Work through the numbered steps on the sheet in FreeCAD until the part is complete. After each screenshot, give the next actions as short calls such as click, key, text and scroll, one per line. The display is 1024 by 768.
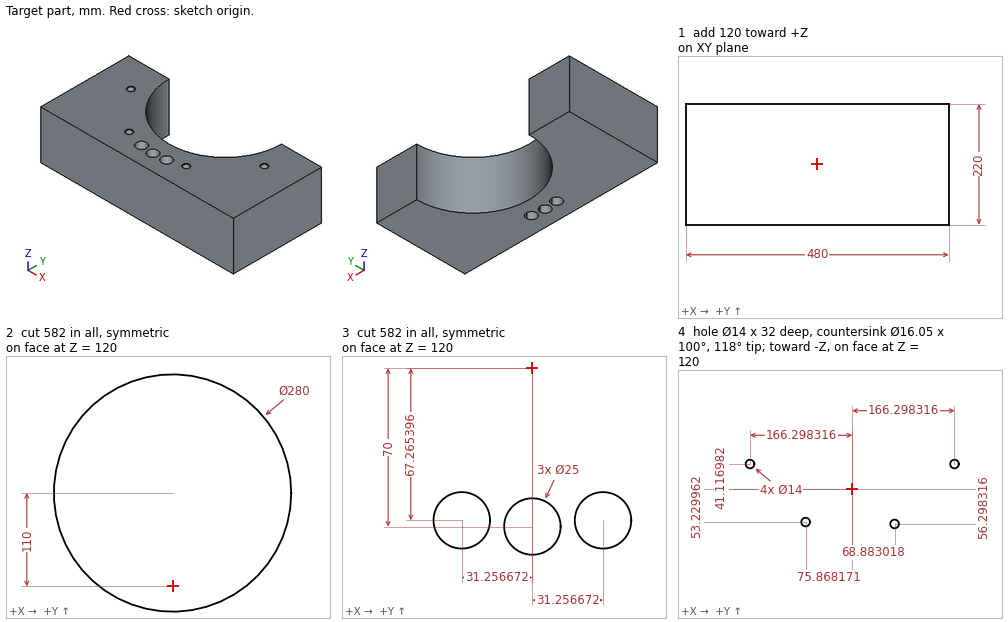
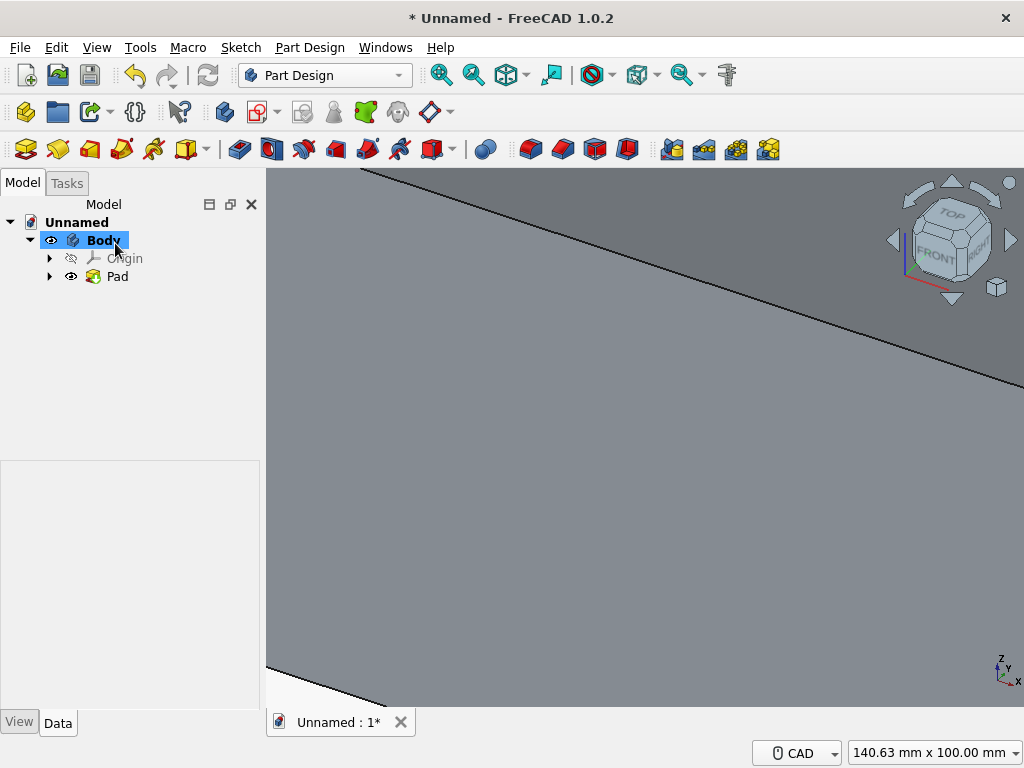
key(v)
key(f)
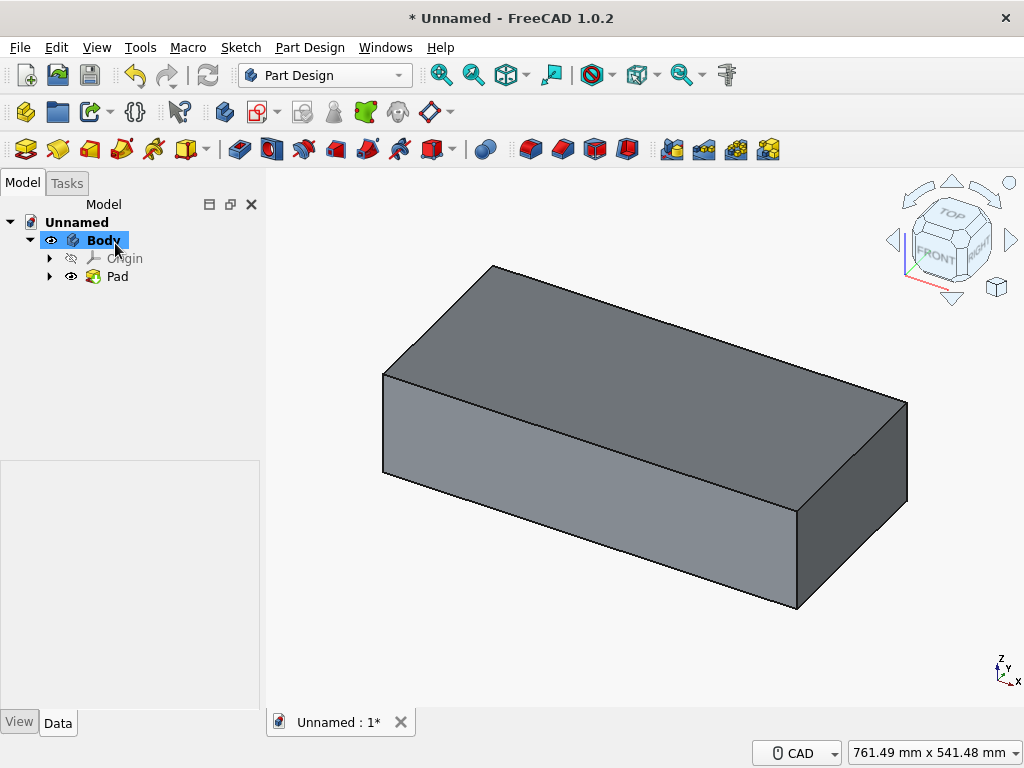
click(704, 407)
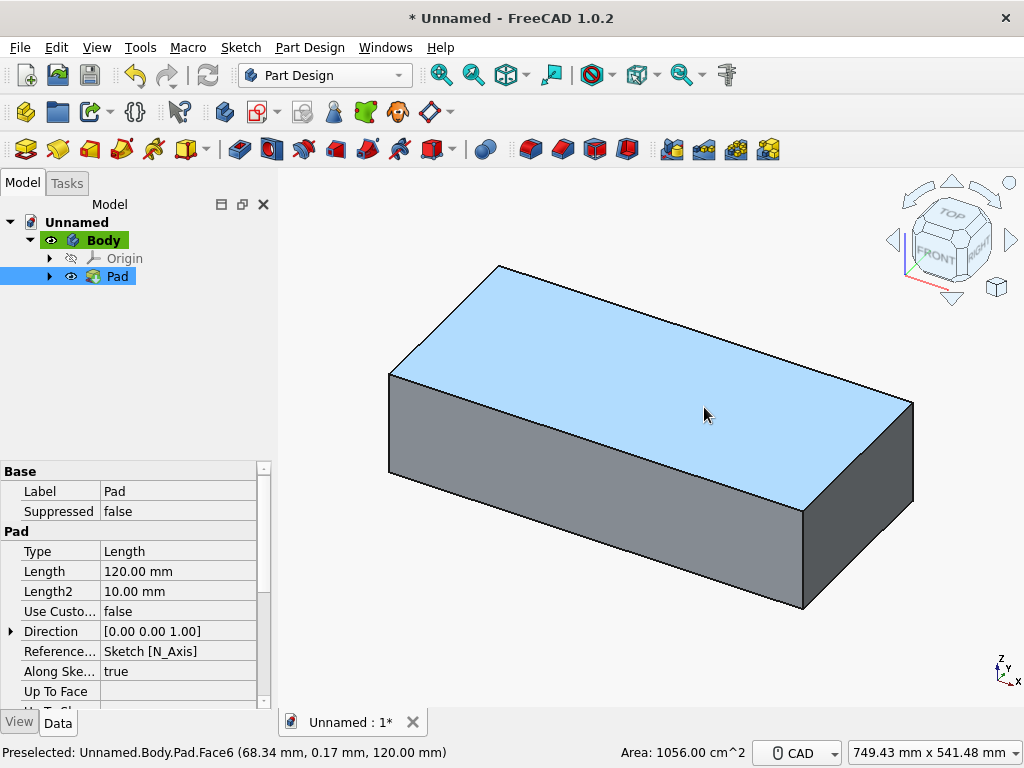
click(258, 112)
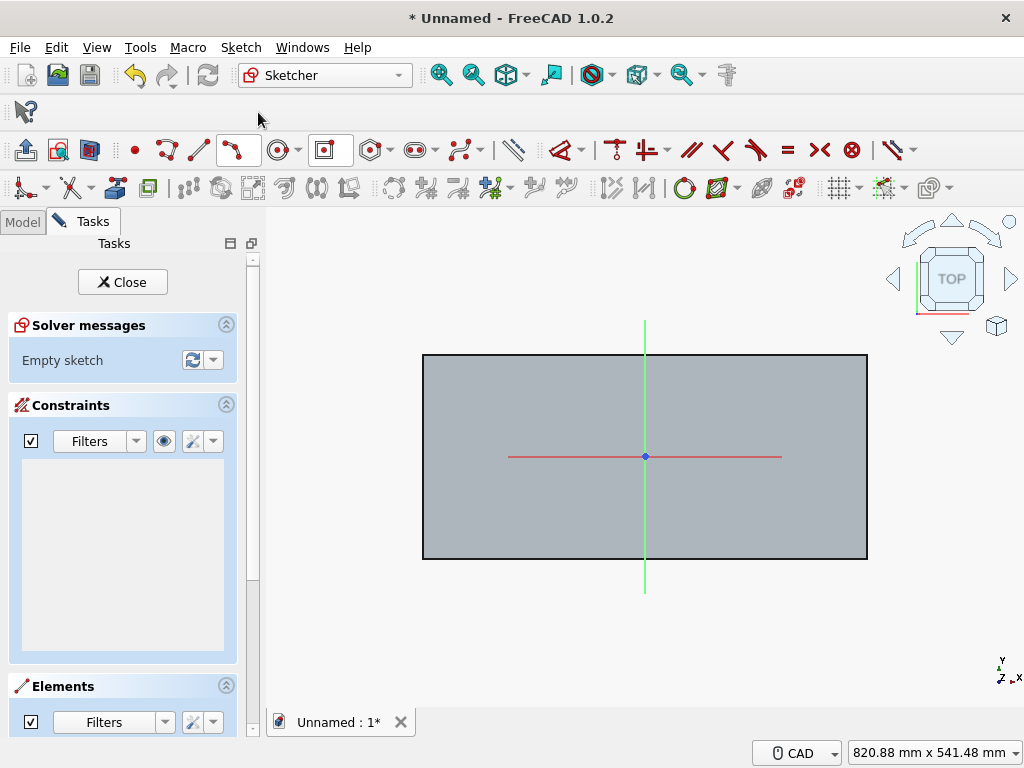
scroll(294, 679, down, 1)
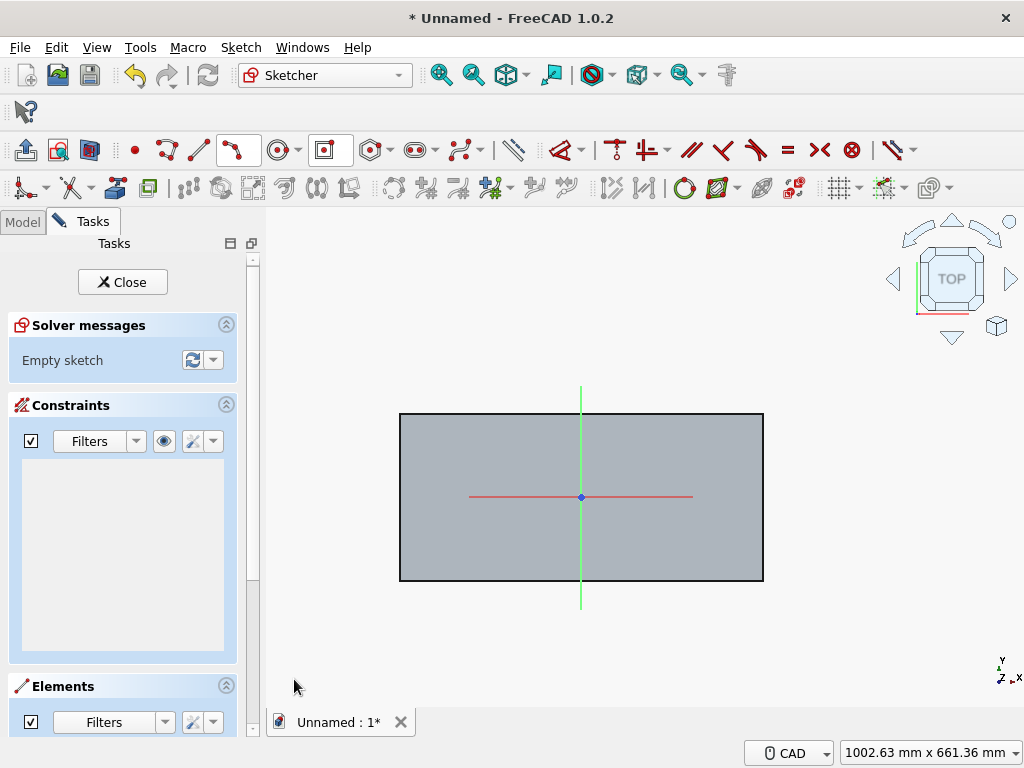
scroll(591, 327, up, 2)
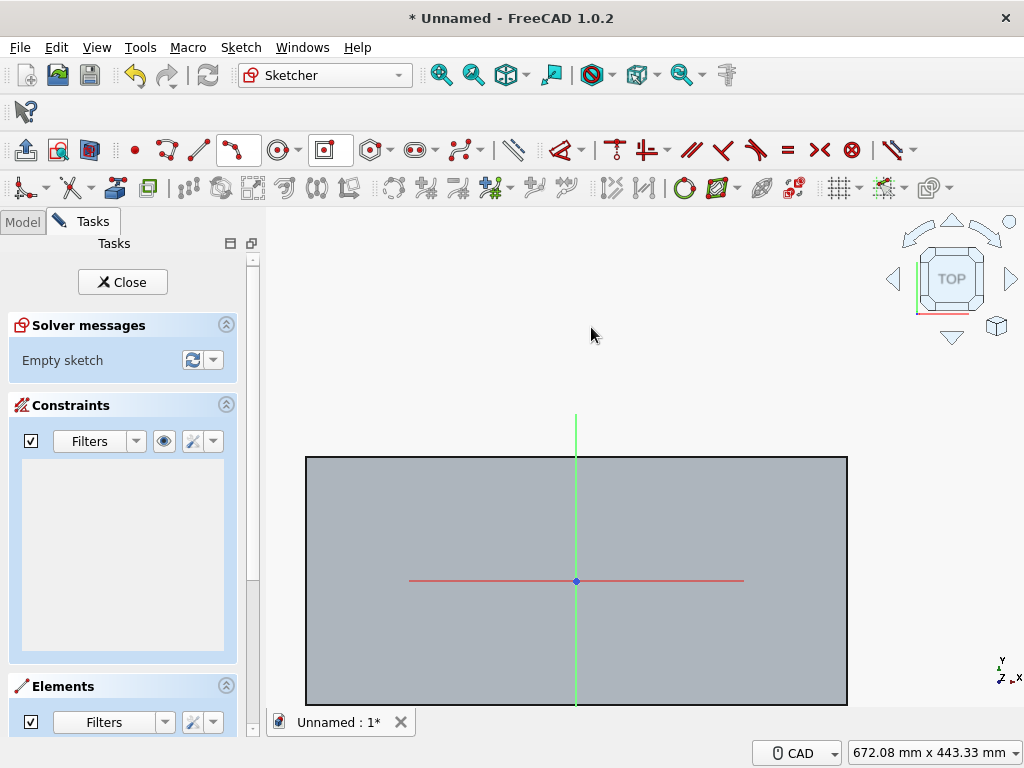
key(g)
key(c)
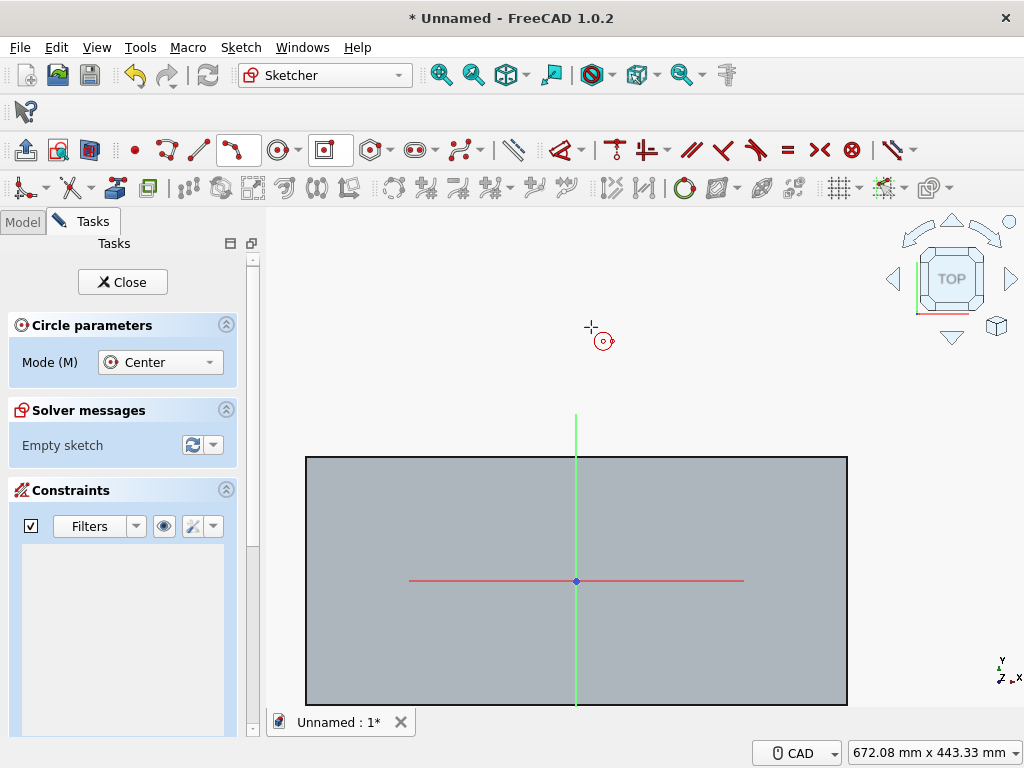
click(576, 457)
move(688, 345)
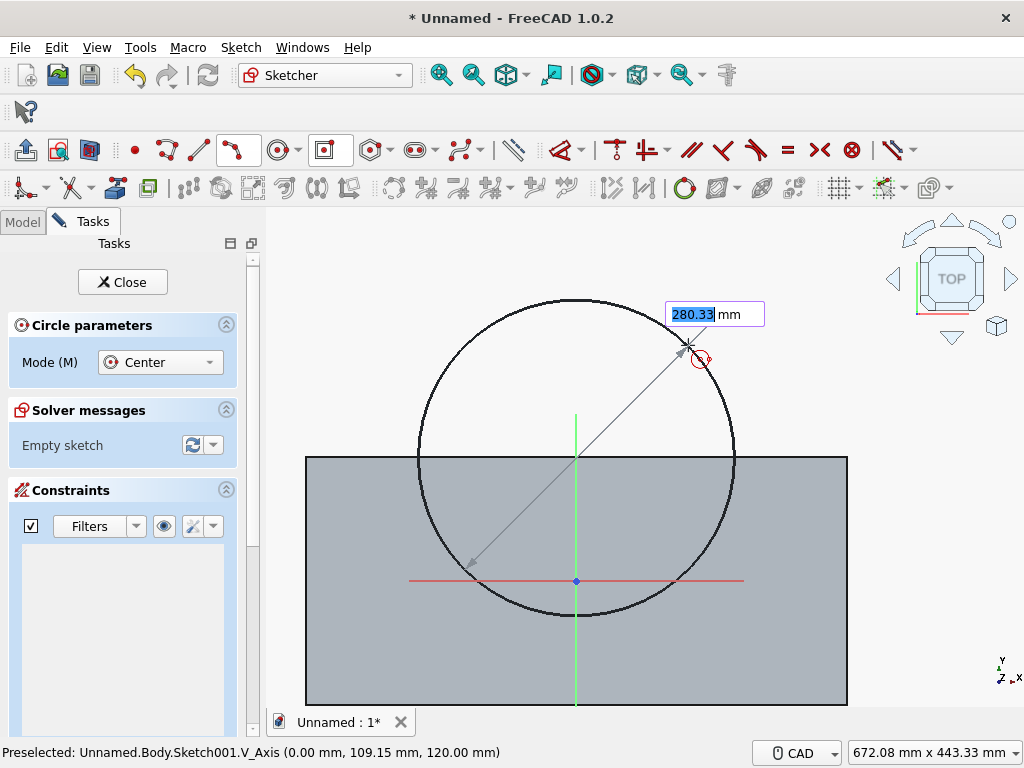
text(280)
key(Return)
key(Escape)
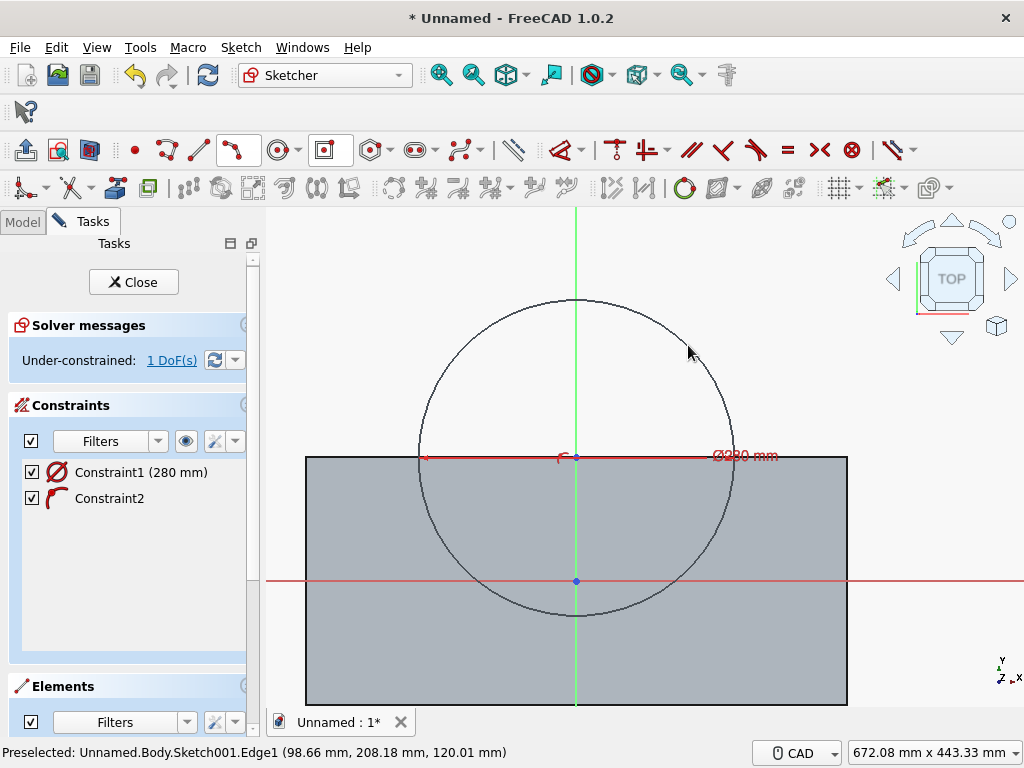
key(d)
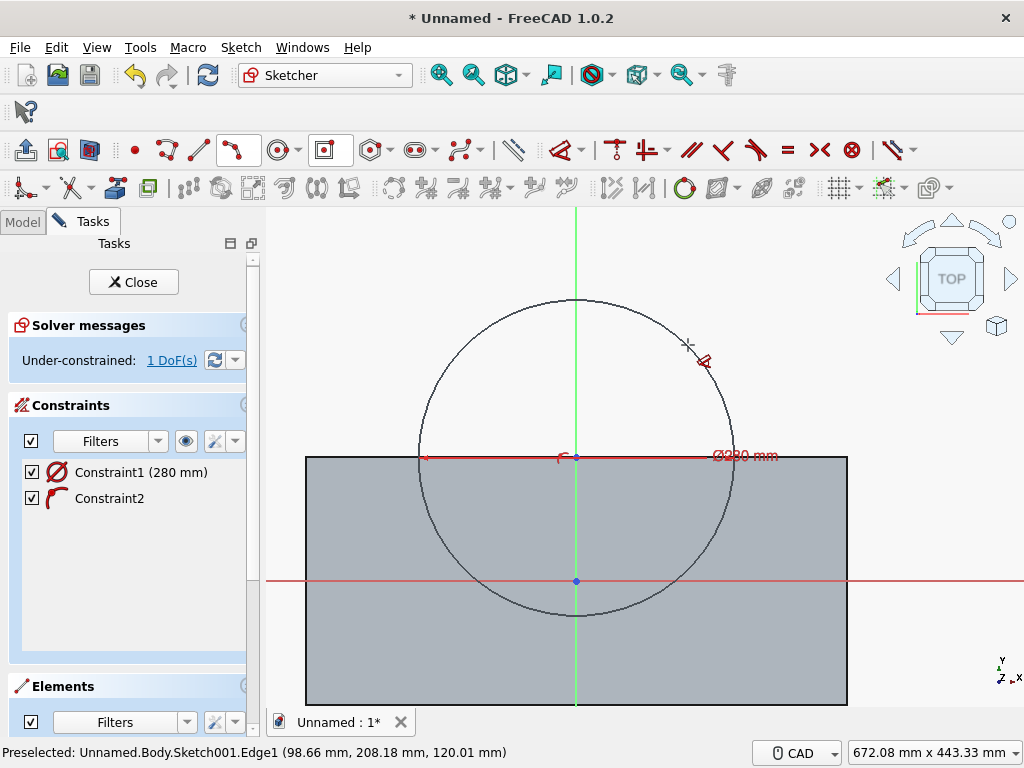
click(576, 458)
click(610, 520)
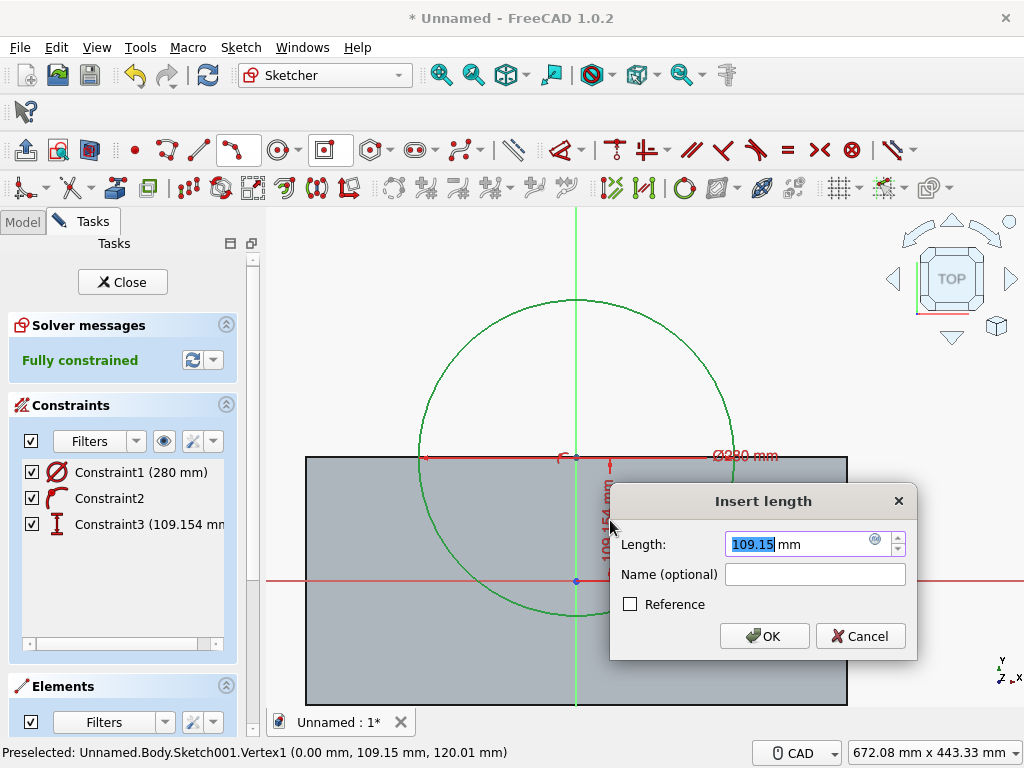
text(110)
key(Return)
key(Escape)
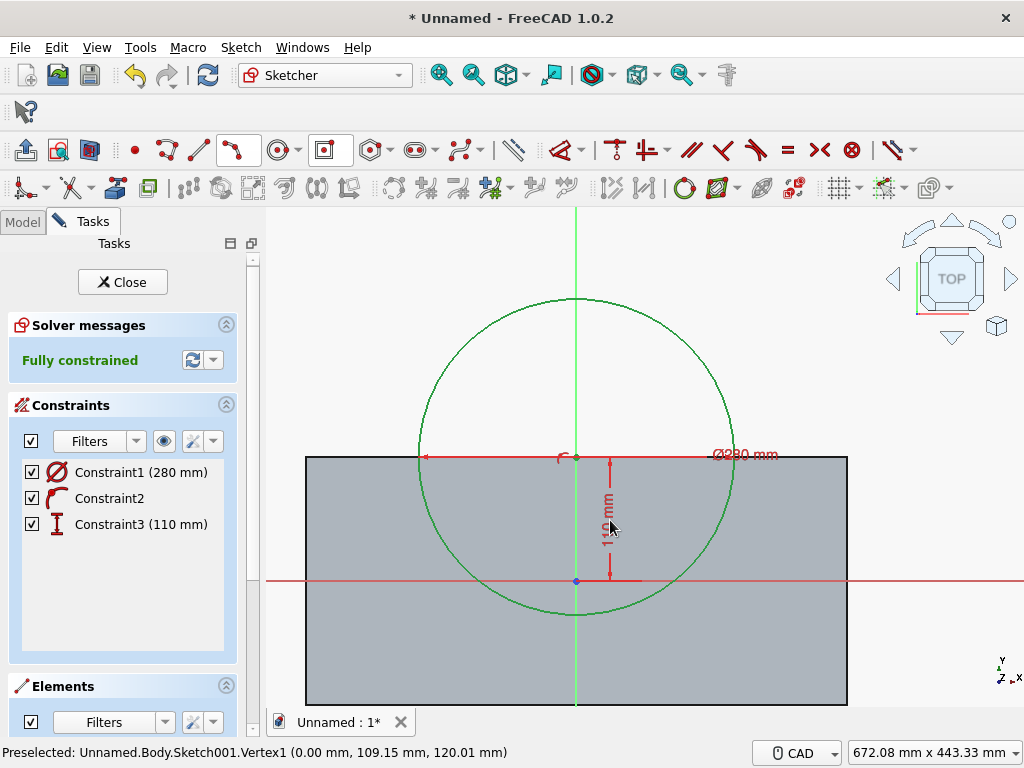
click(123, 282)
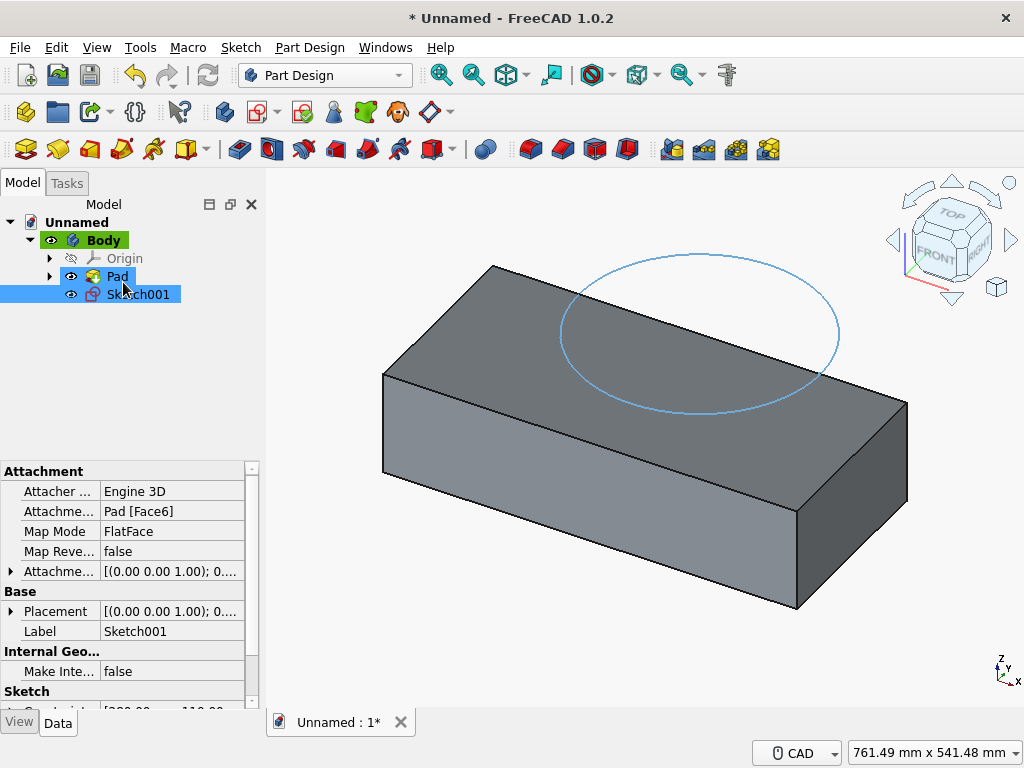
click(240, 150)